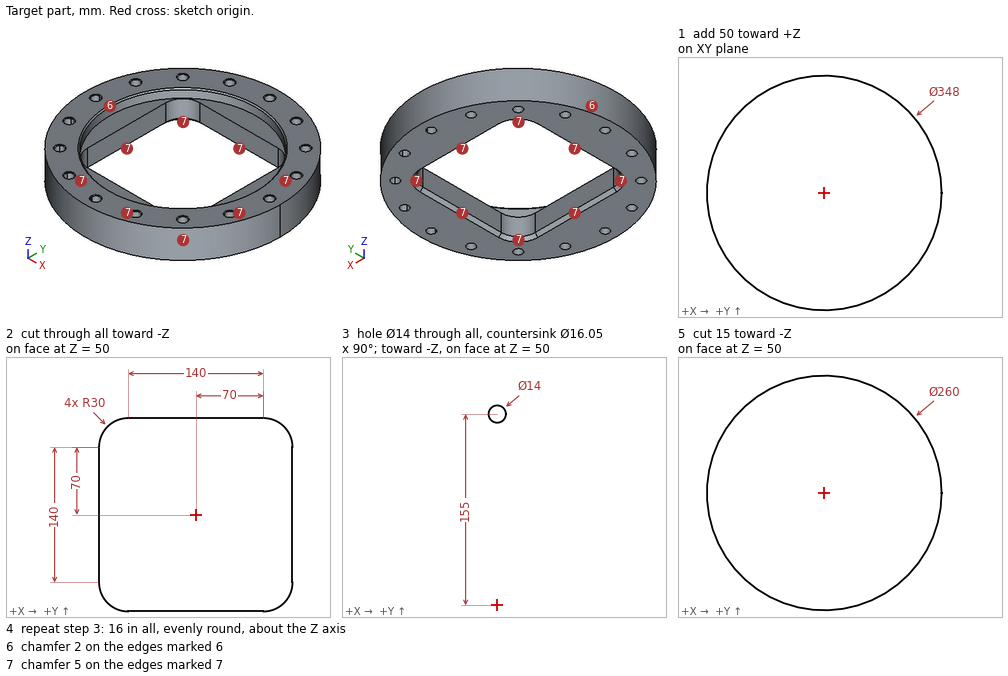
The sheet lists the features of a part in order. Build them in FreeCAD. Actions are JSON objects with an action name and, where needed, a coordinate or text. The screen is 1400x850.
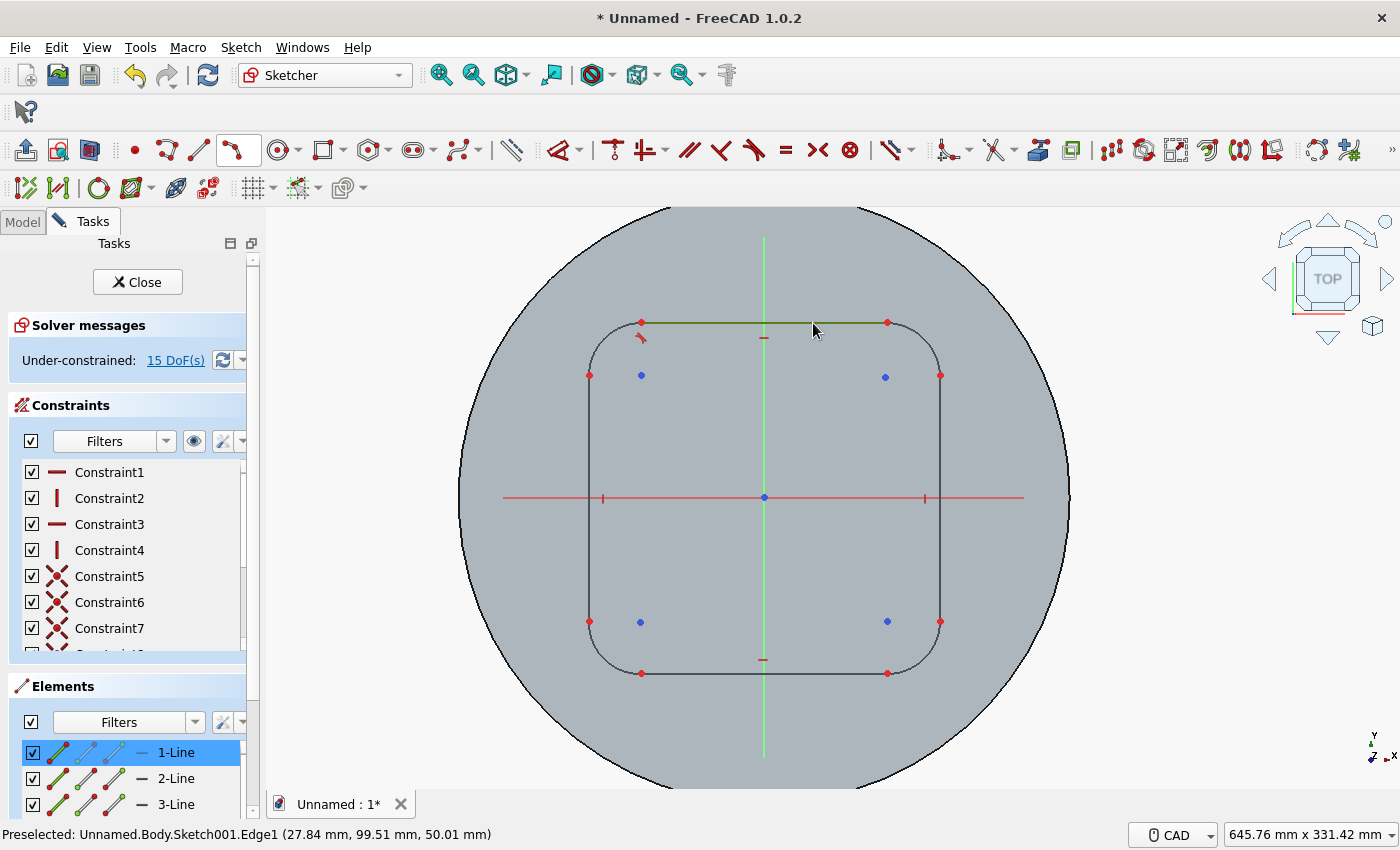
{"action": "left_click", "coordinate": [934, 352]}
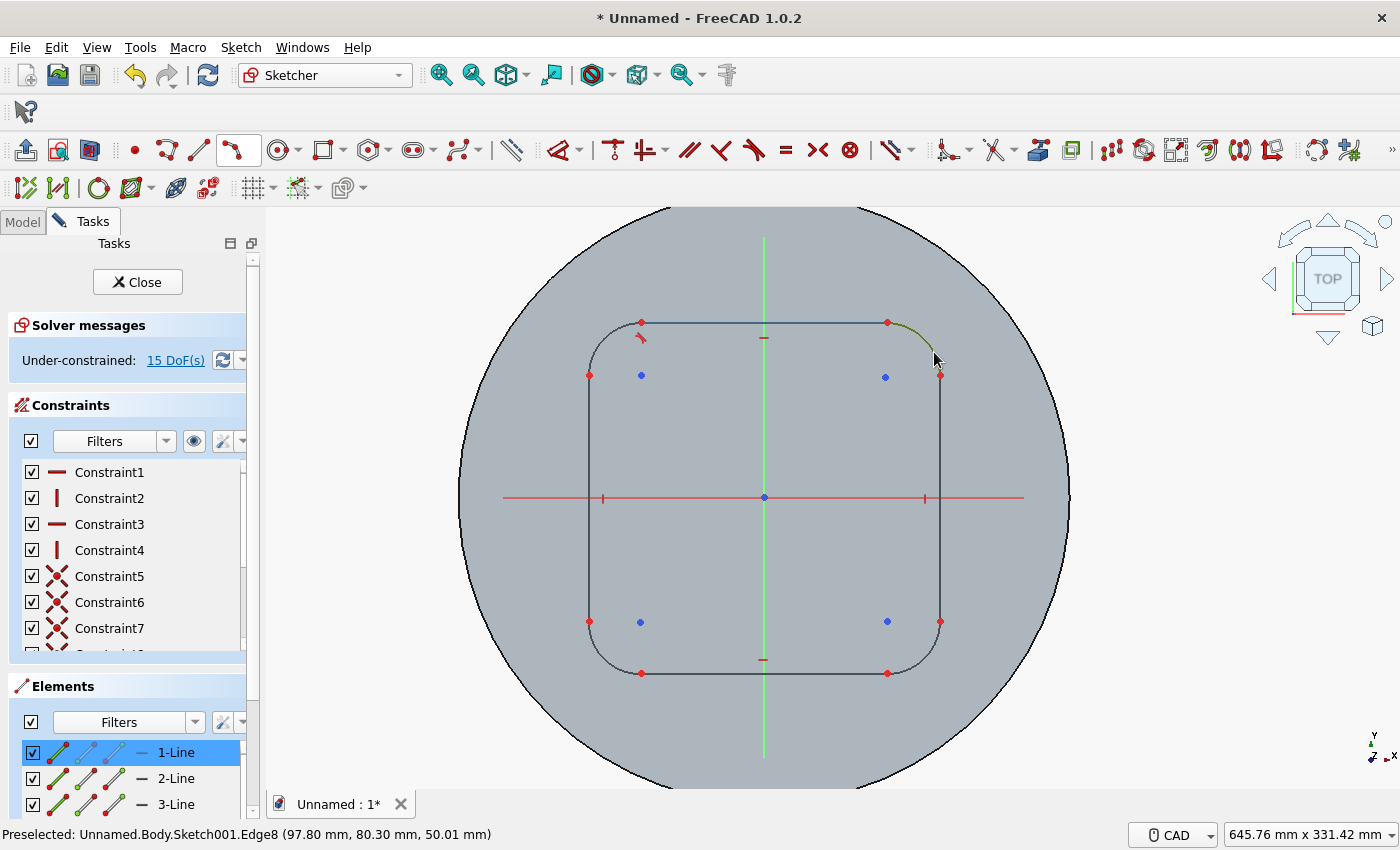
{"action": "left_click", "coordinate": [754, 150]}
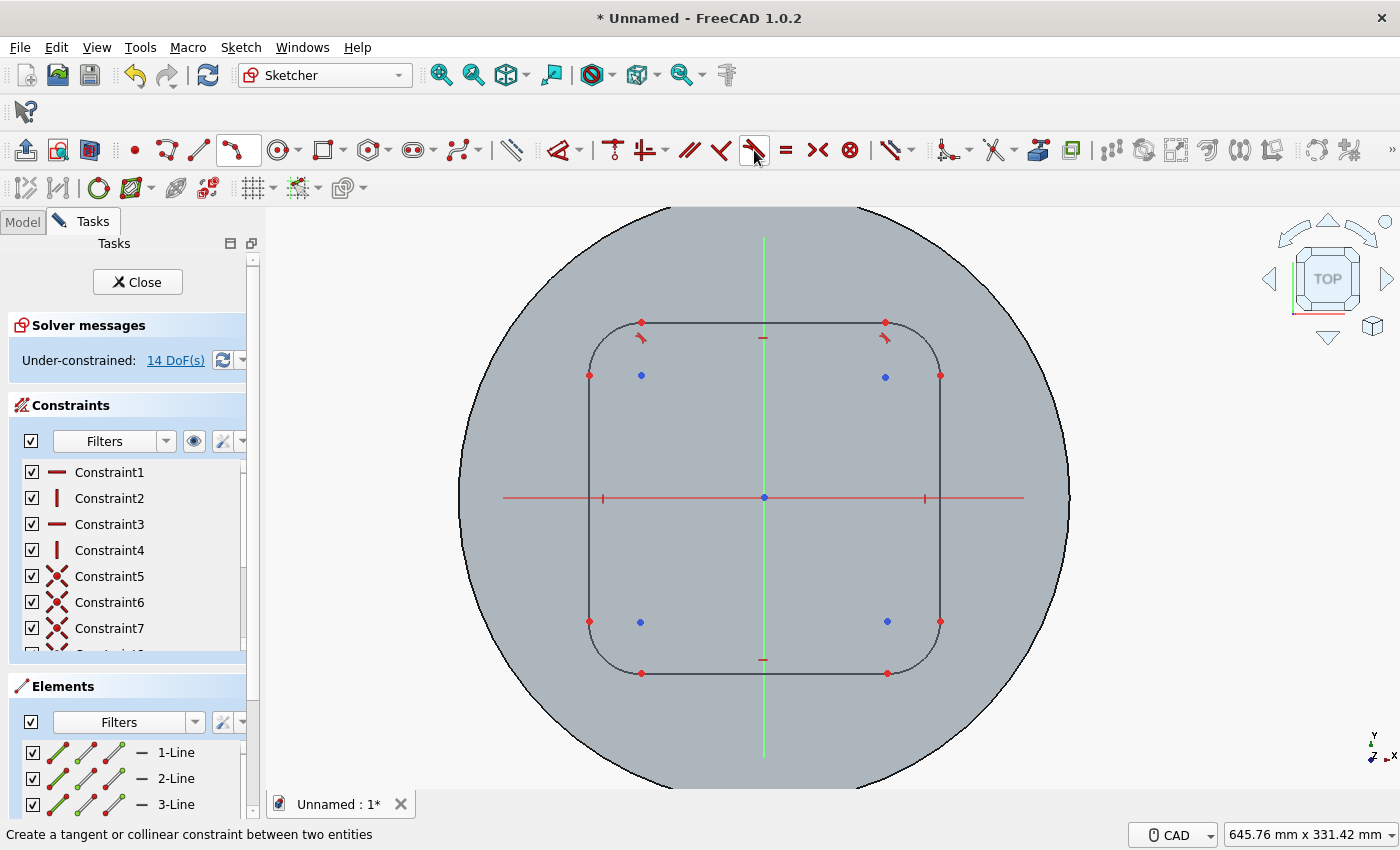
{"action": "left_click", "coordinate": [589, 450]}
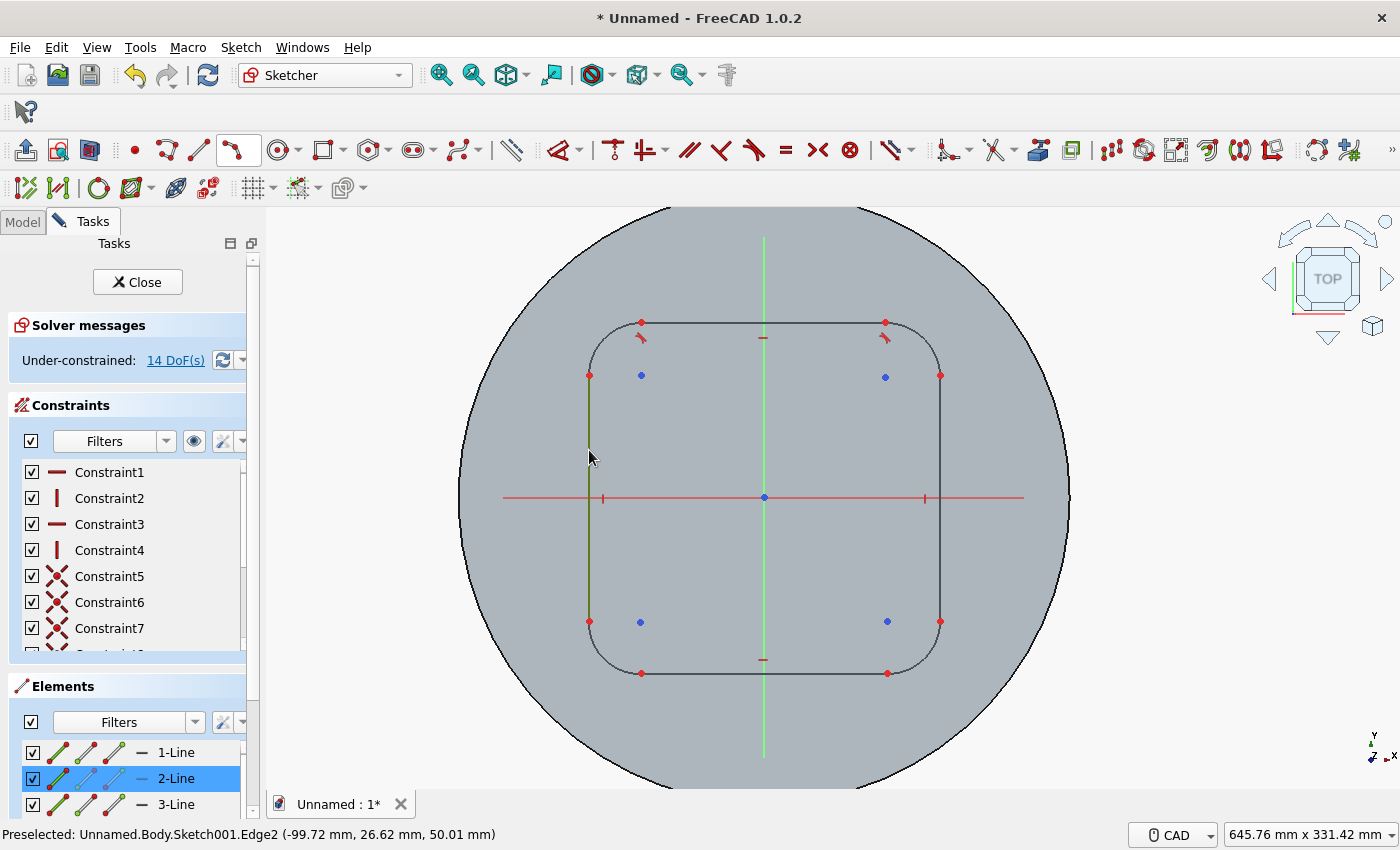
{"action": "left_click", "coordinate": [618, 329]}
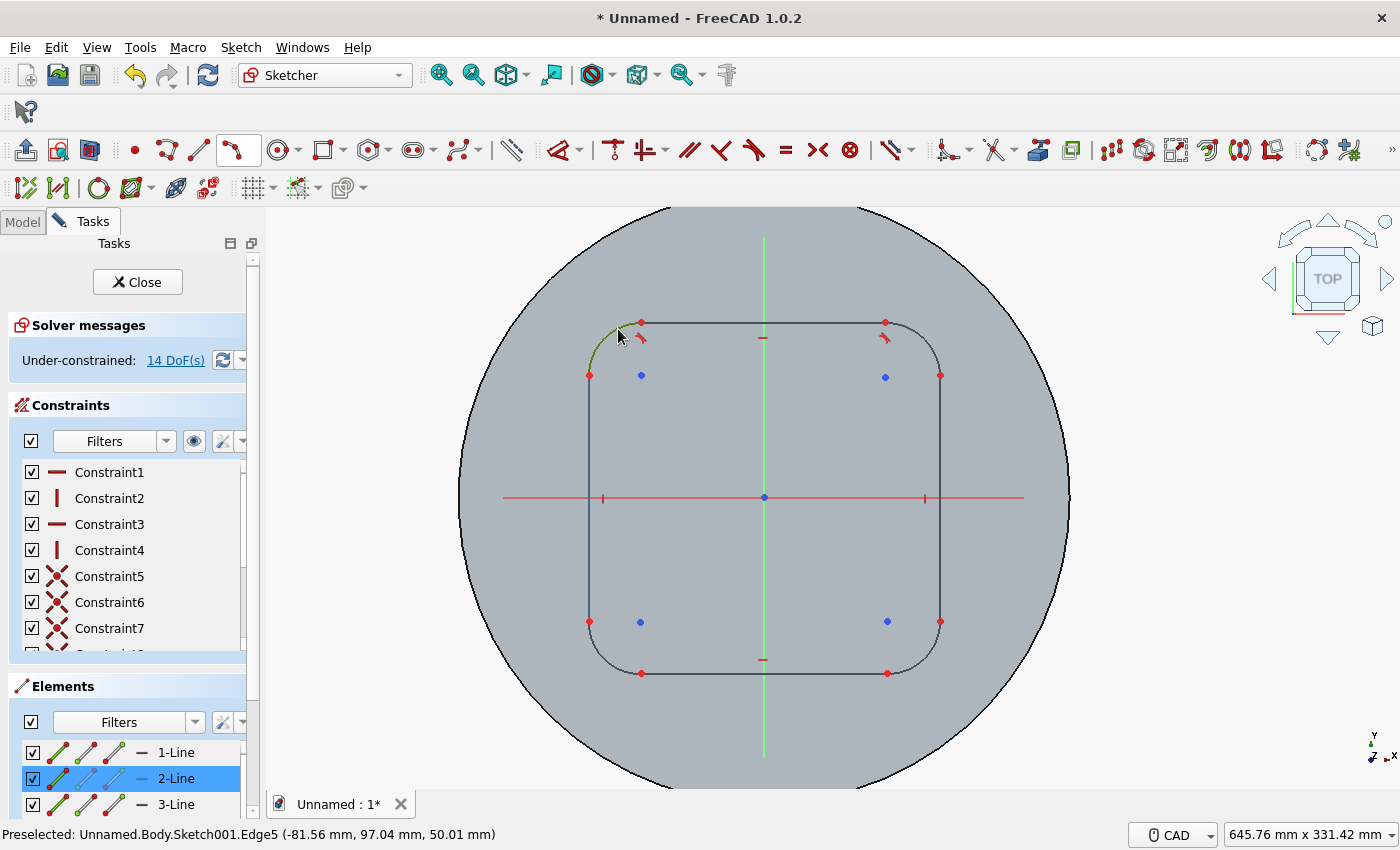
{"action": "left_click", "coordinate": [754, 150]}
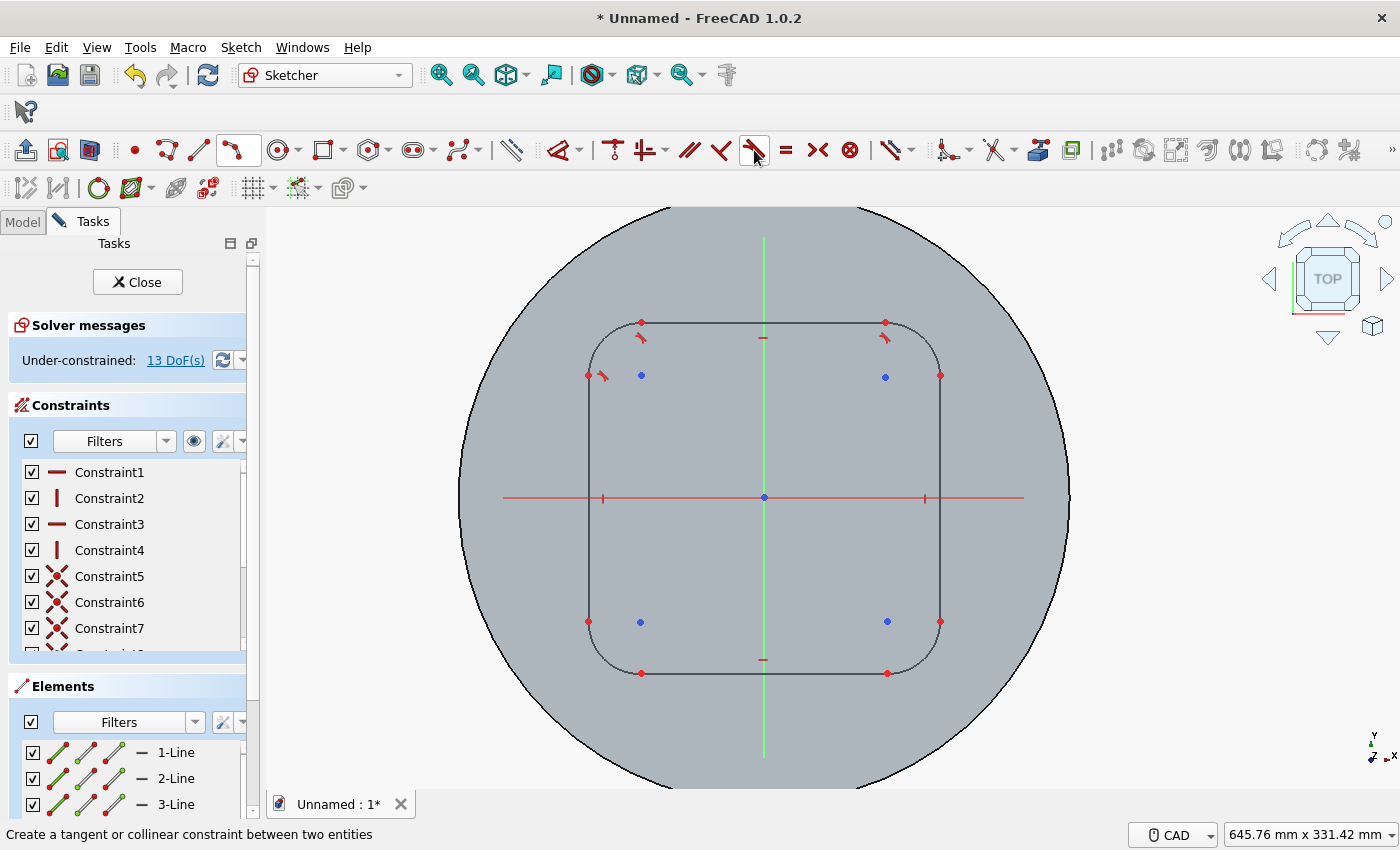
{"action": "left_click", "coordinate": [589, 450]}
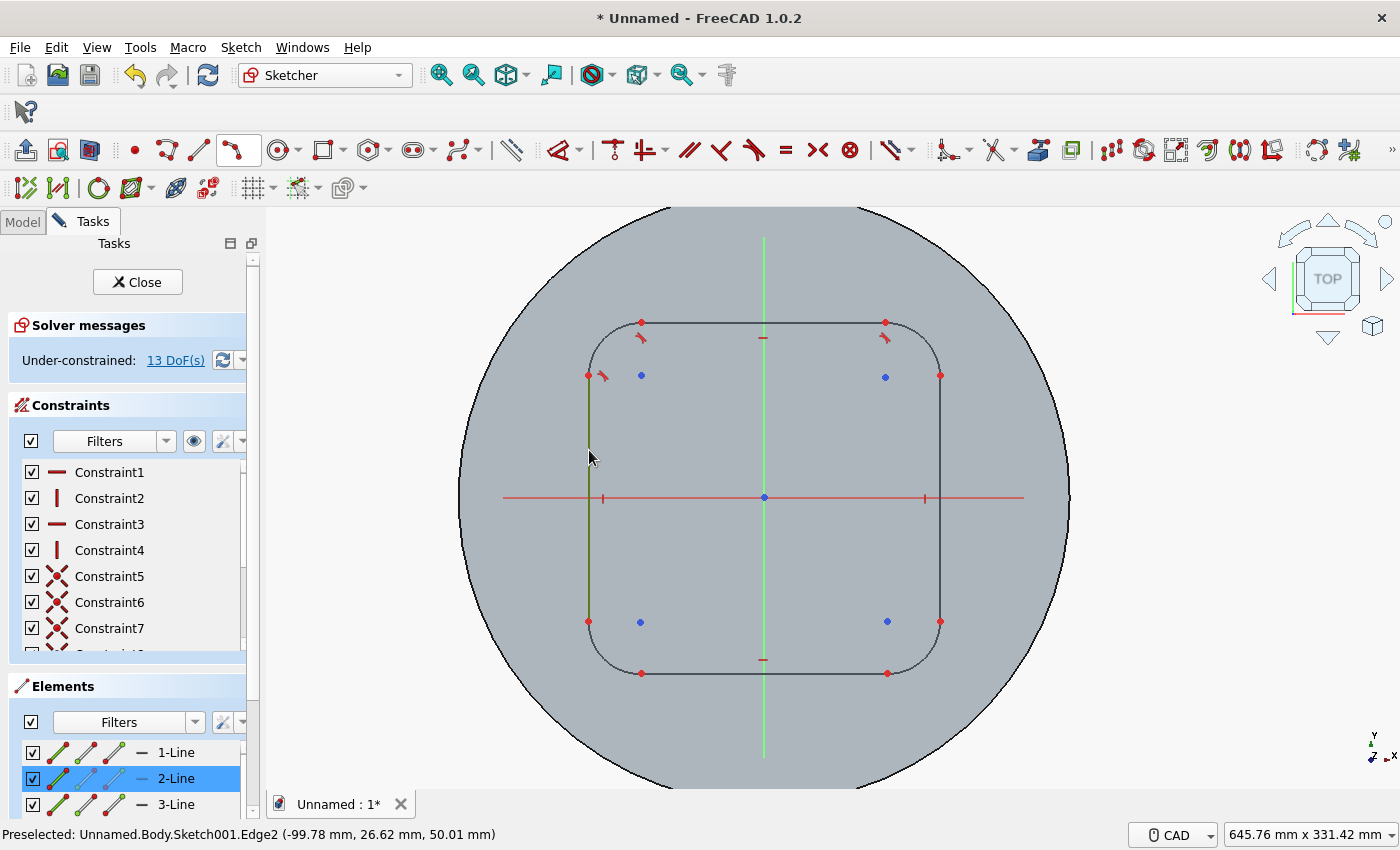
{"action": "left_click", "coordinate": [594, 646]}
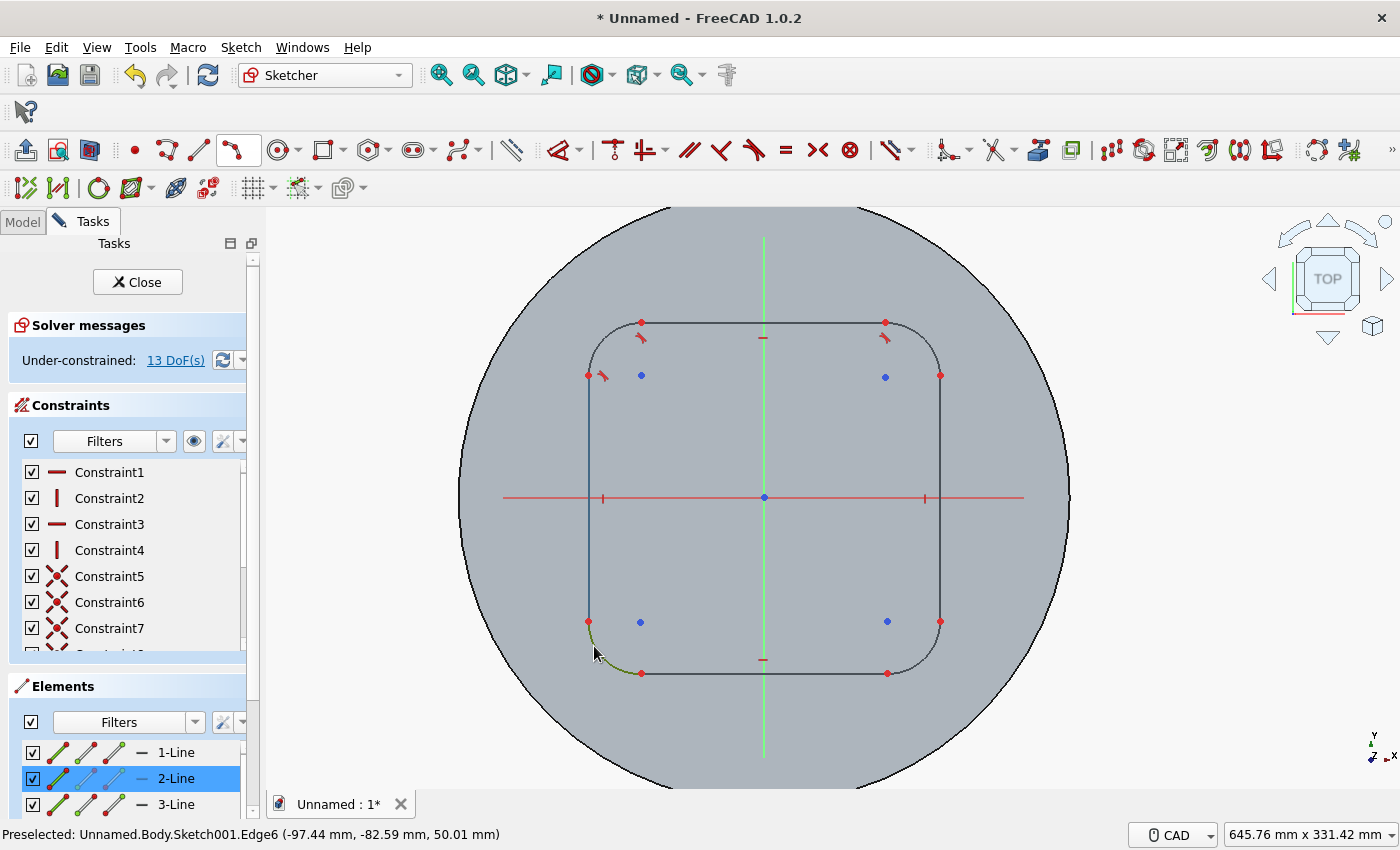
{"action": "left_click", "coordinate": [754, 150]}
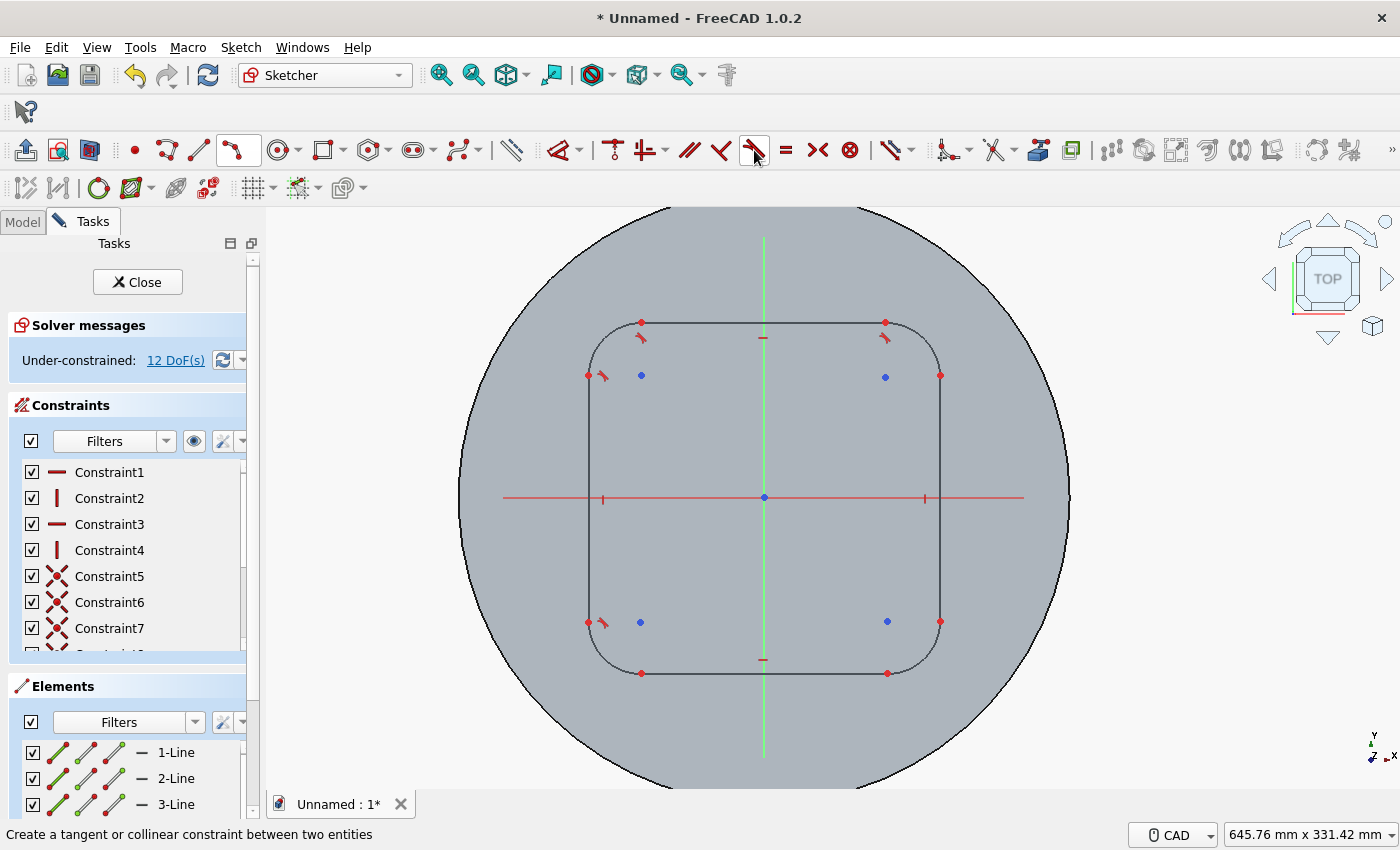
{"action": "left_click", "coordinate": [715, 674]}